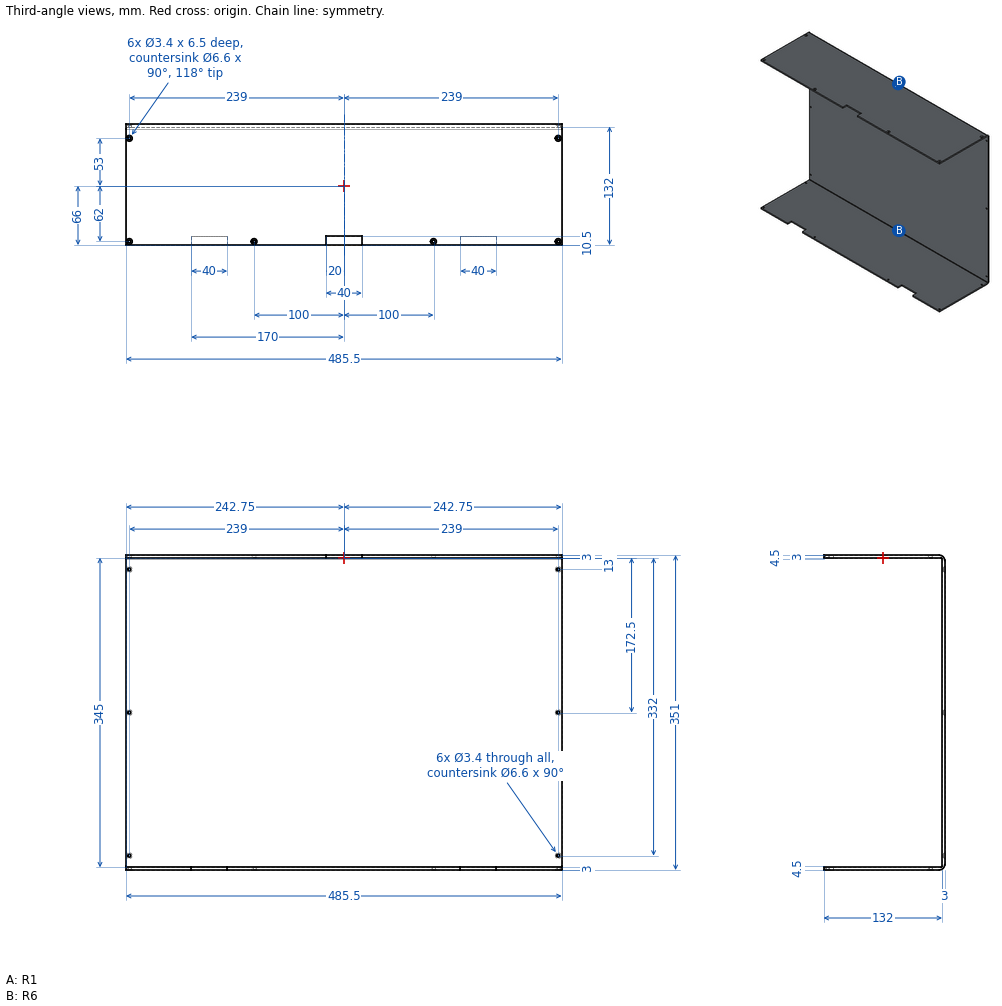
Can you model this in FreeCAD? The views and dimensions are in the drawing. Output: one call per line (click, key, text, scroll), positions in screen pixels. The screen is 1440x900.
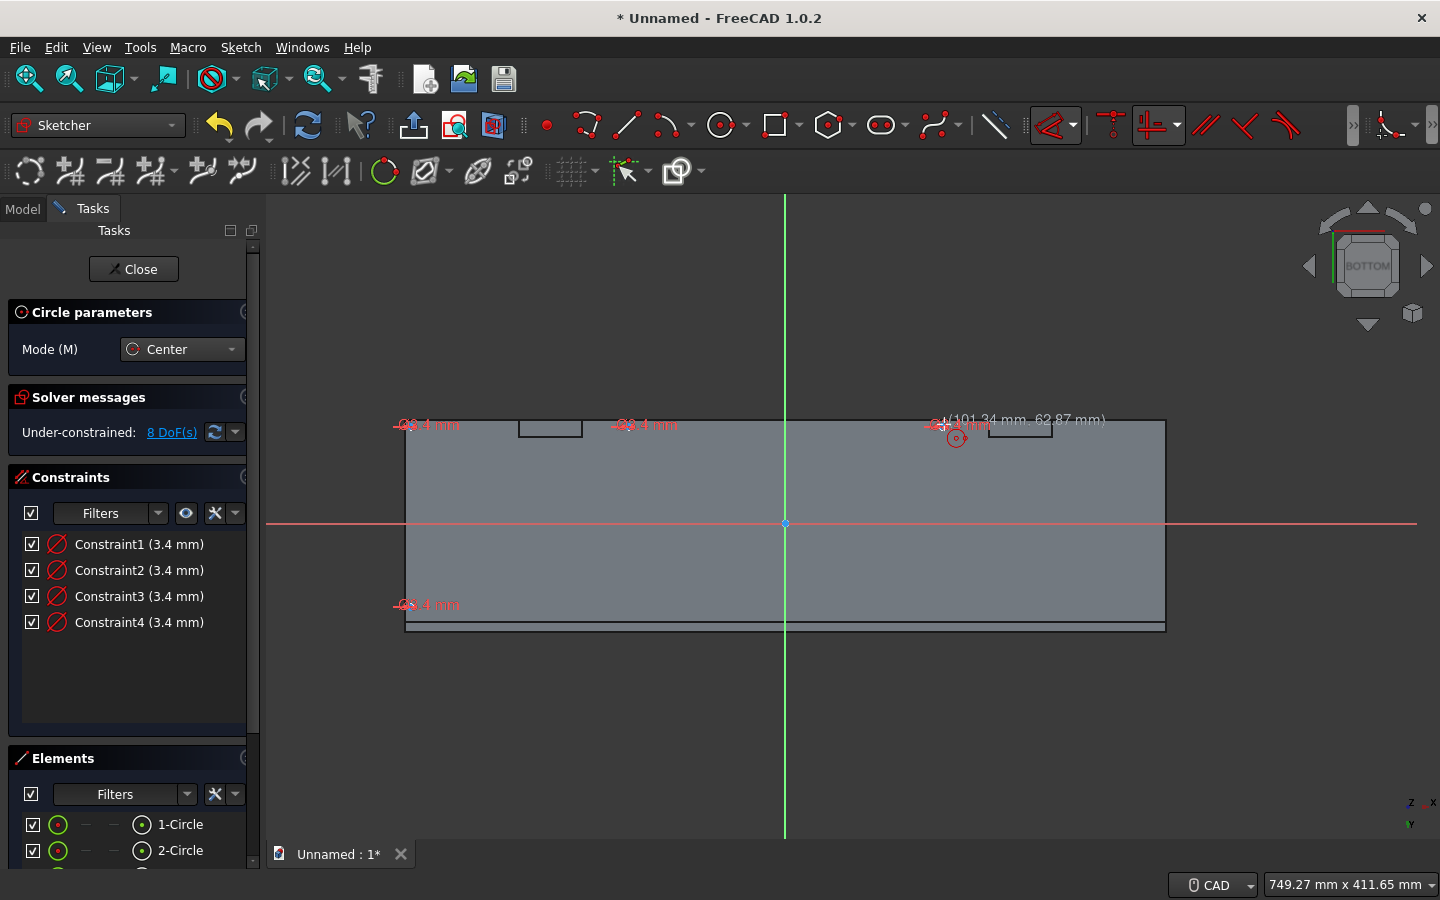
scroll(1160, 426, up, 11)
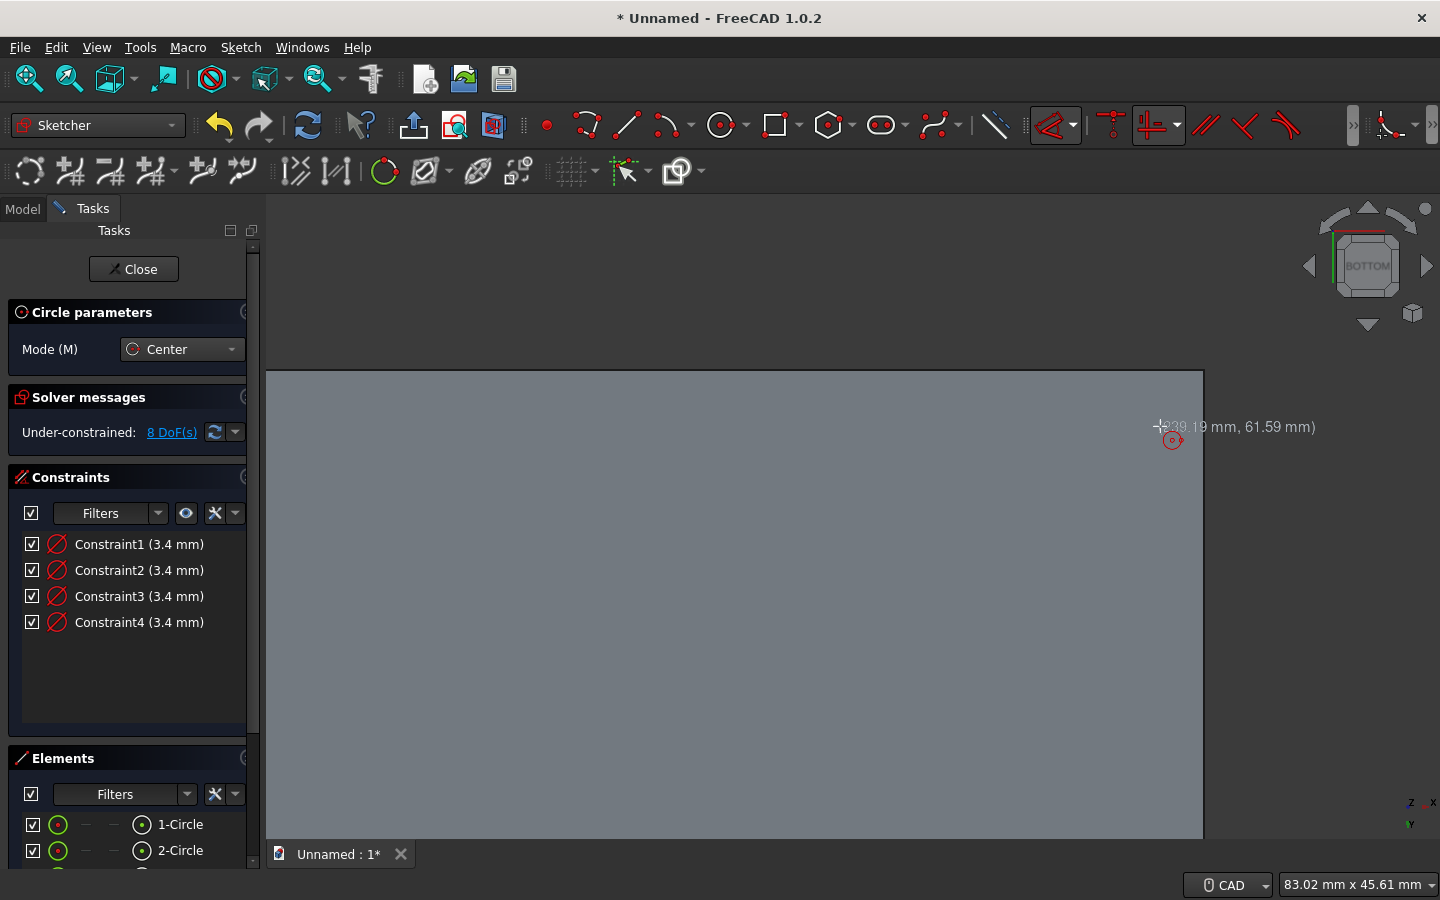
scroll(1160, 426, down, 11)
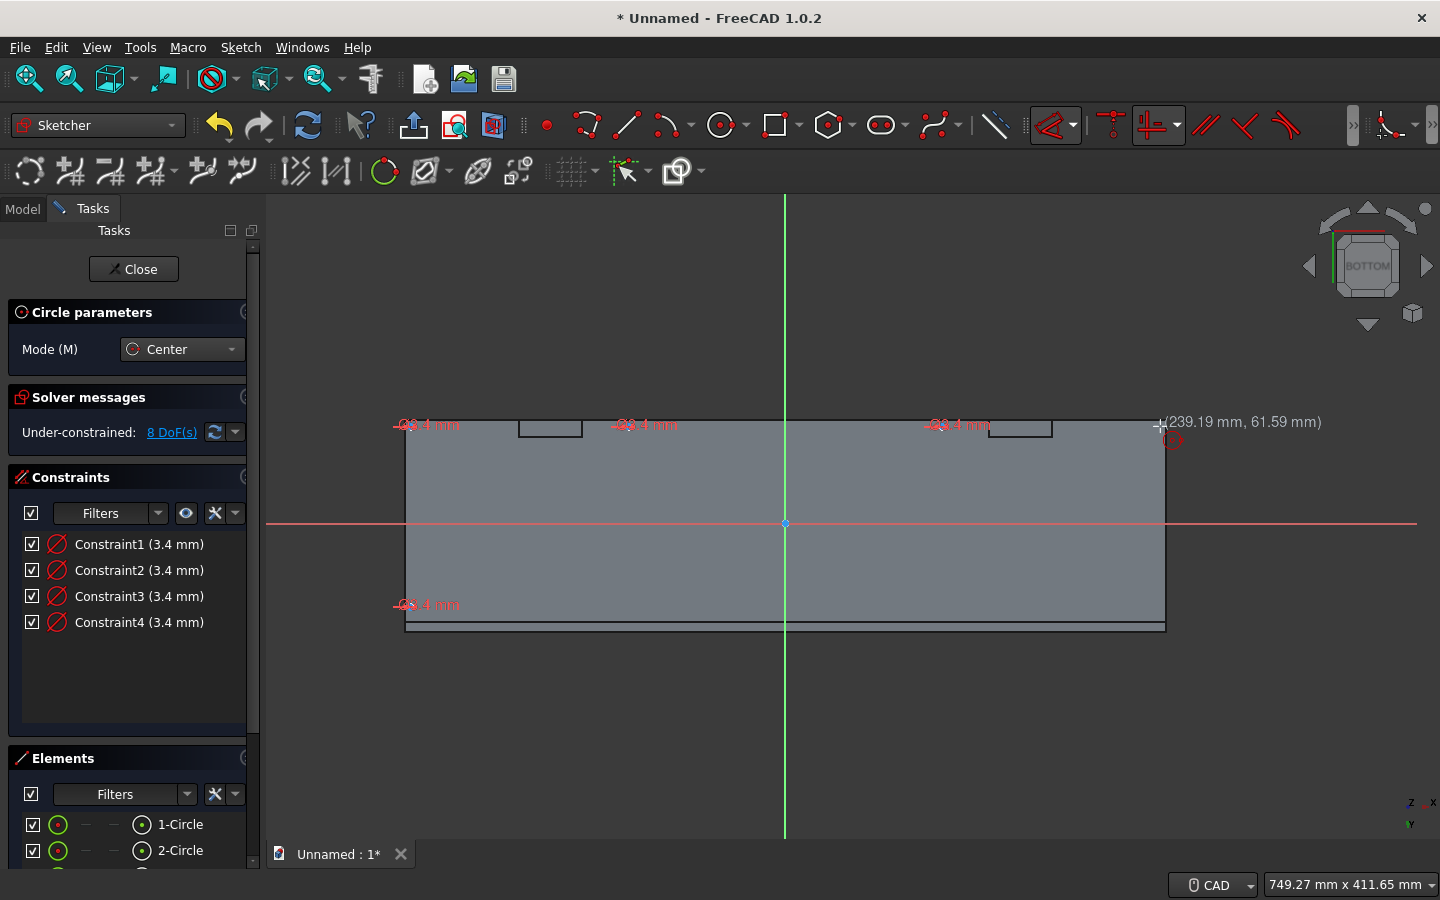
click(1160, 426)
move(1162, 424)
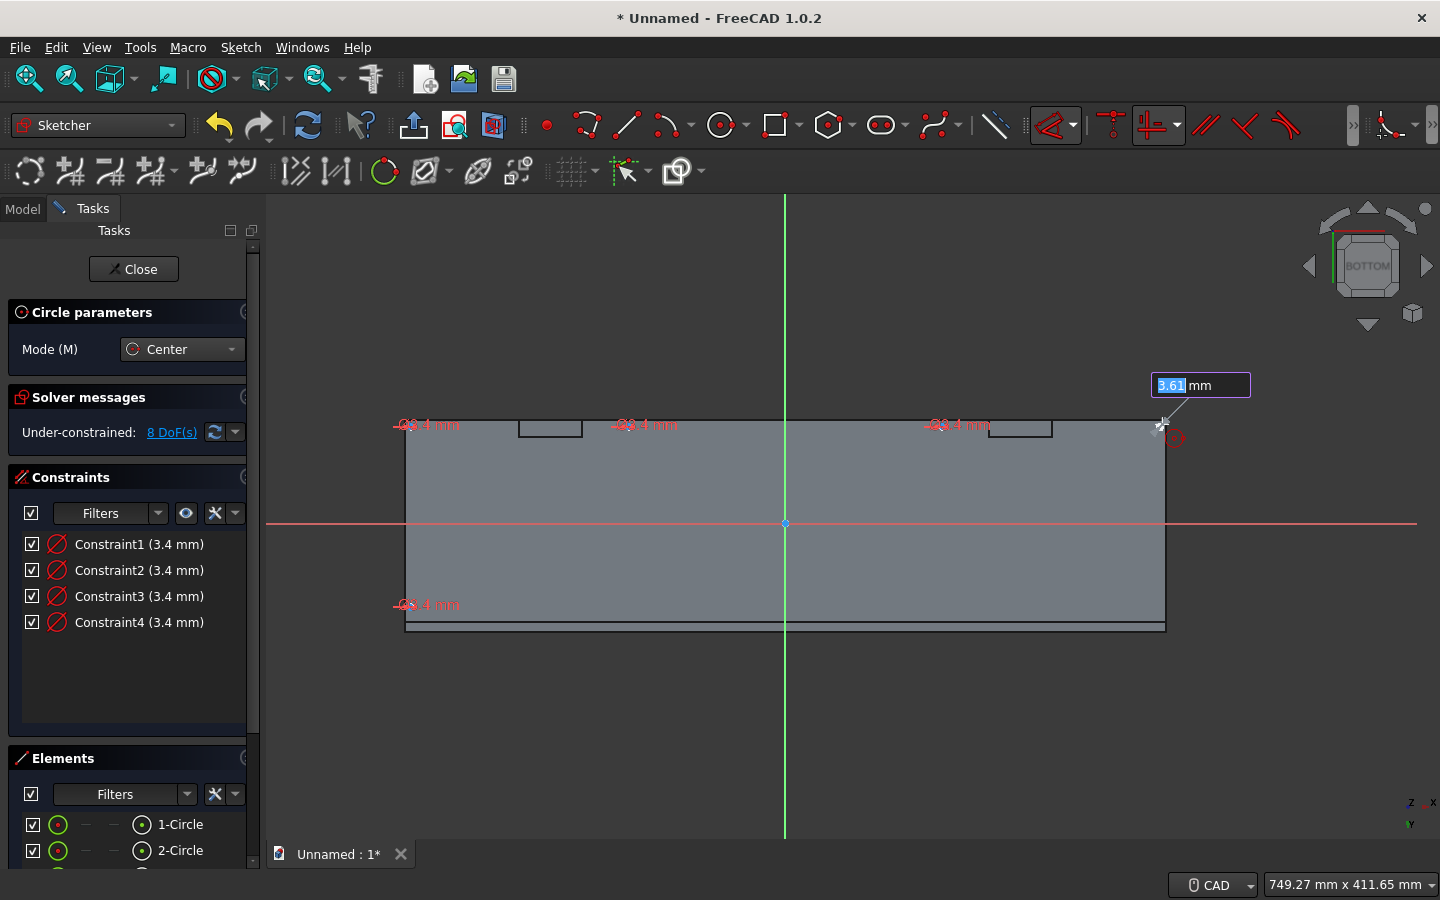
text(3.4)
key(Return)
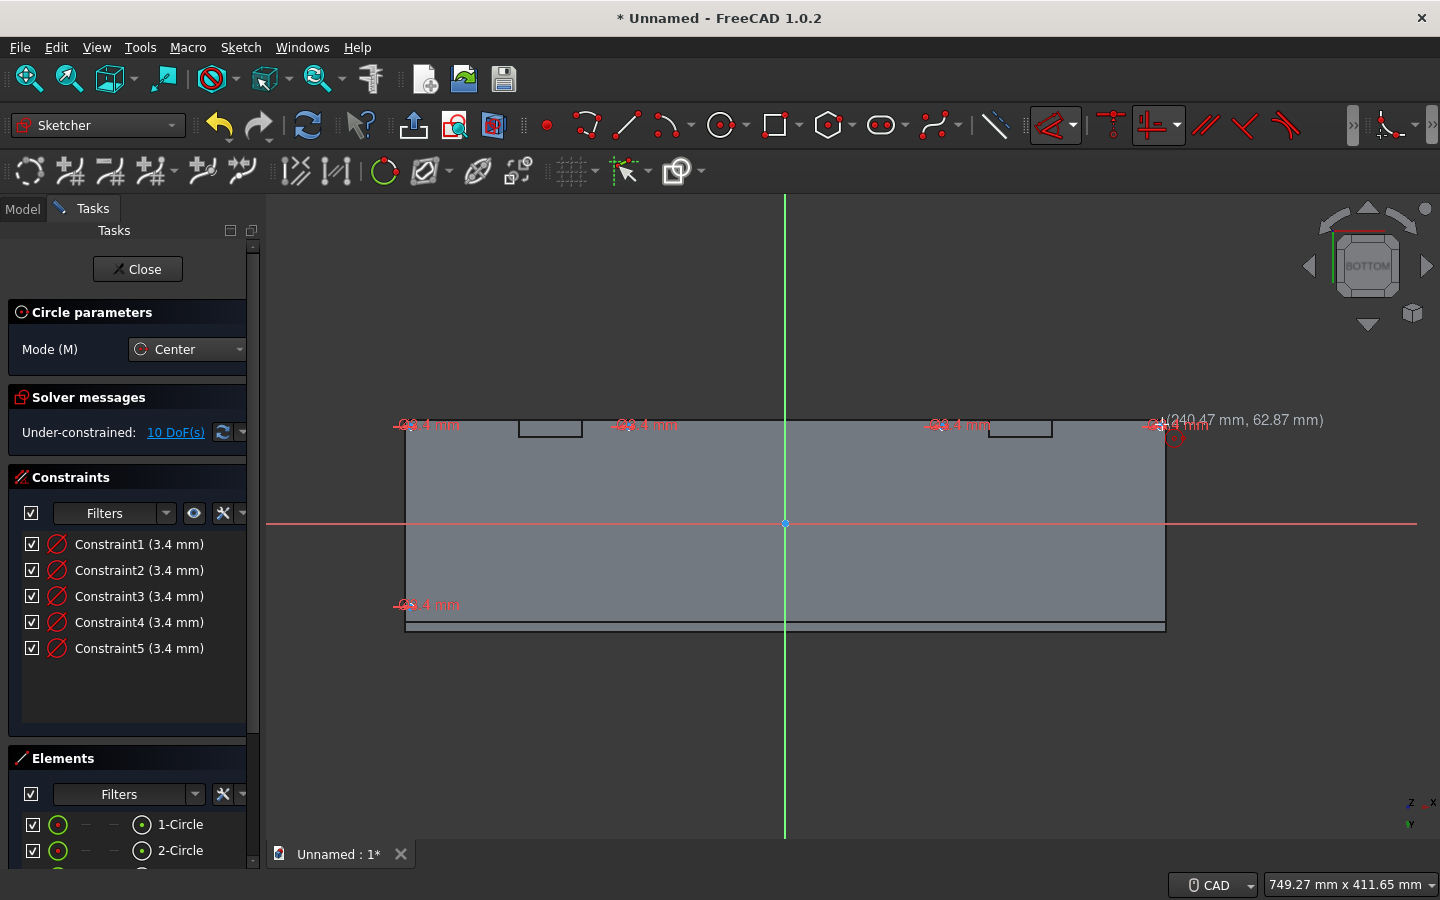
scroll(1160, 607, up, 11)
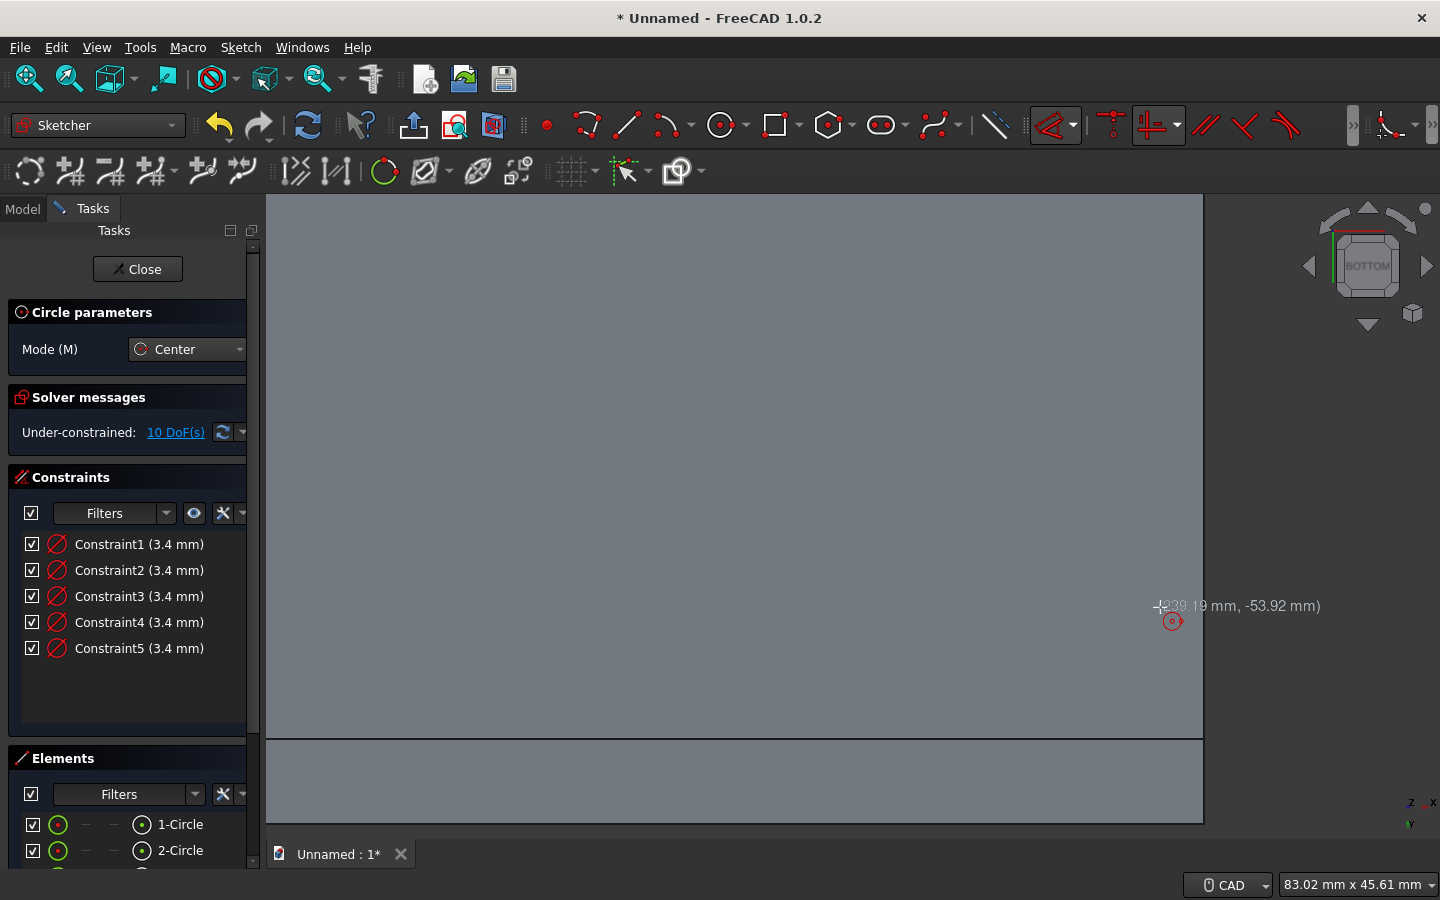
scroll(1160, 608, down, 11)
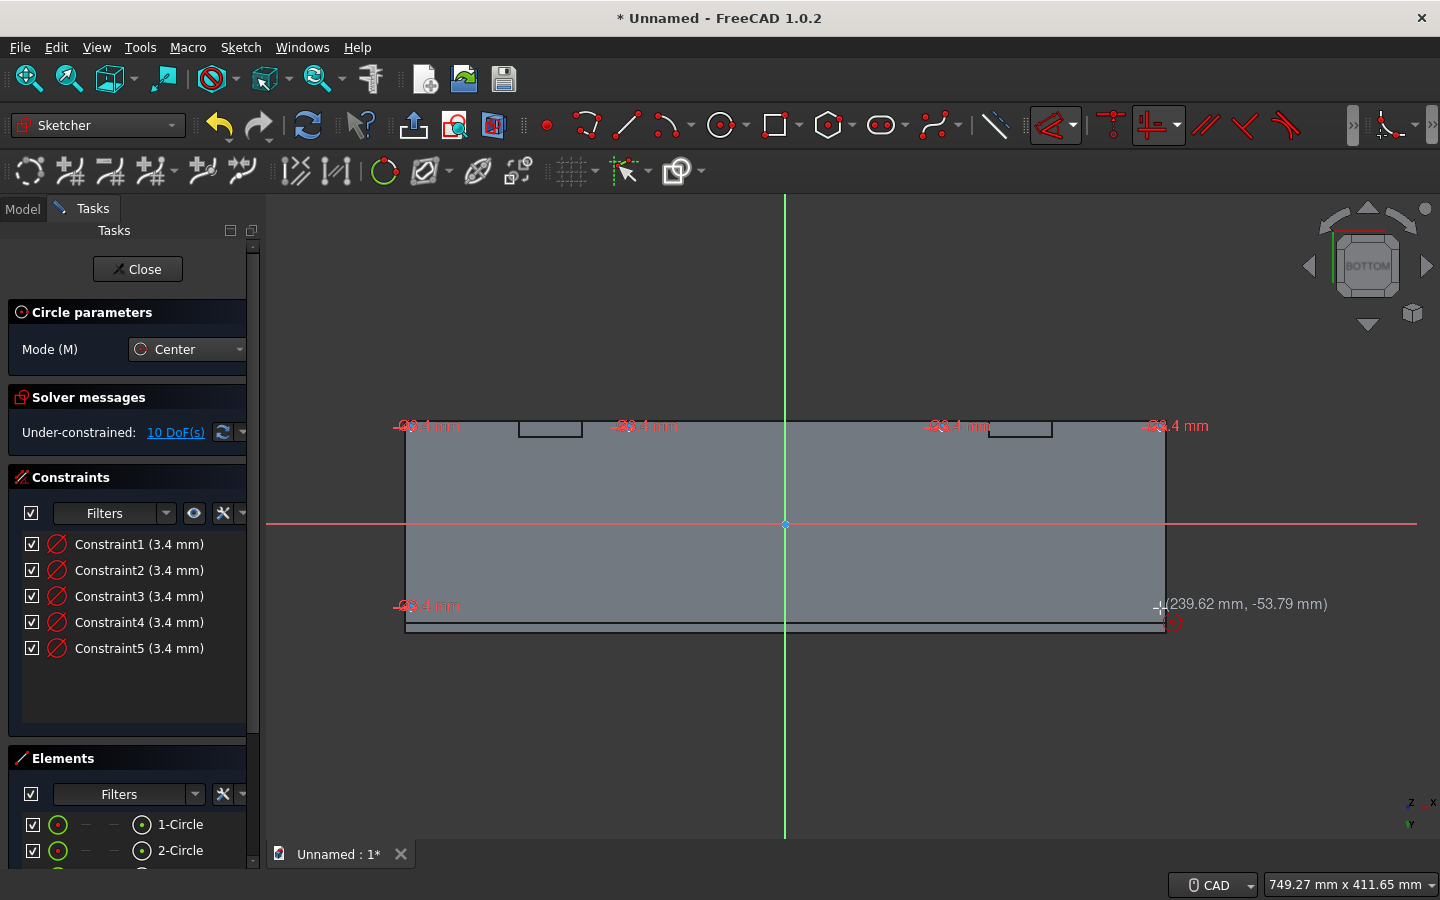
click(1160, 607)
move(1162, 606)